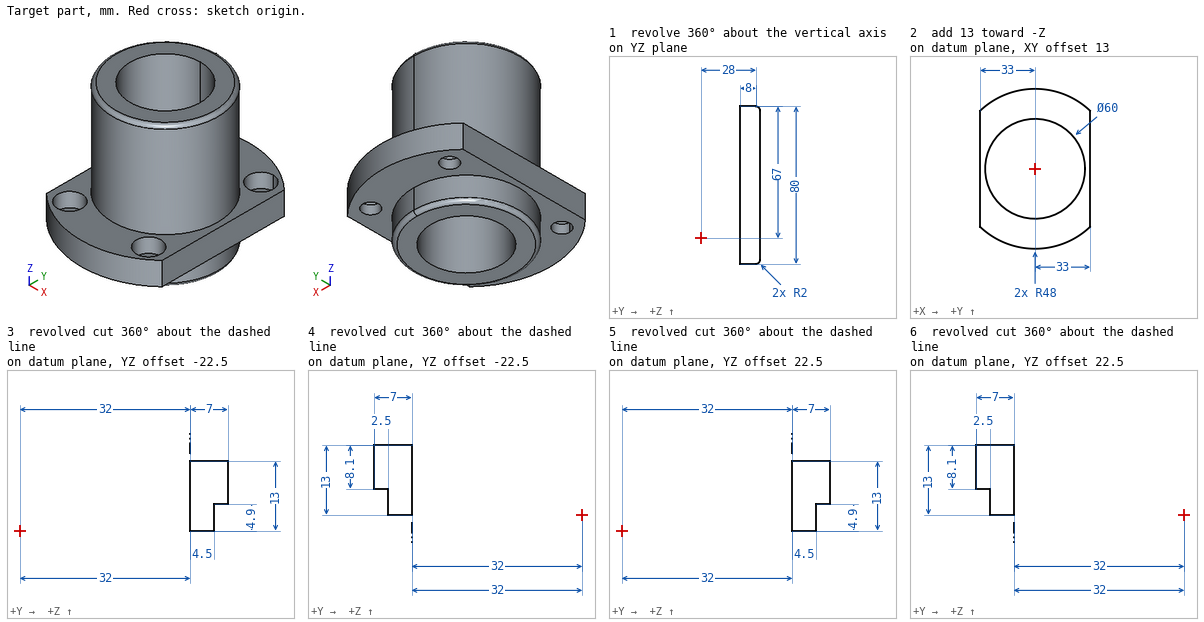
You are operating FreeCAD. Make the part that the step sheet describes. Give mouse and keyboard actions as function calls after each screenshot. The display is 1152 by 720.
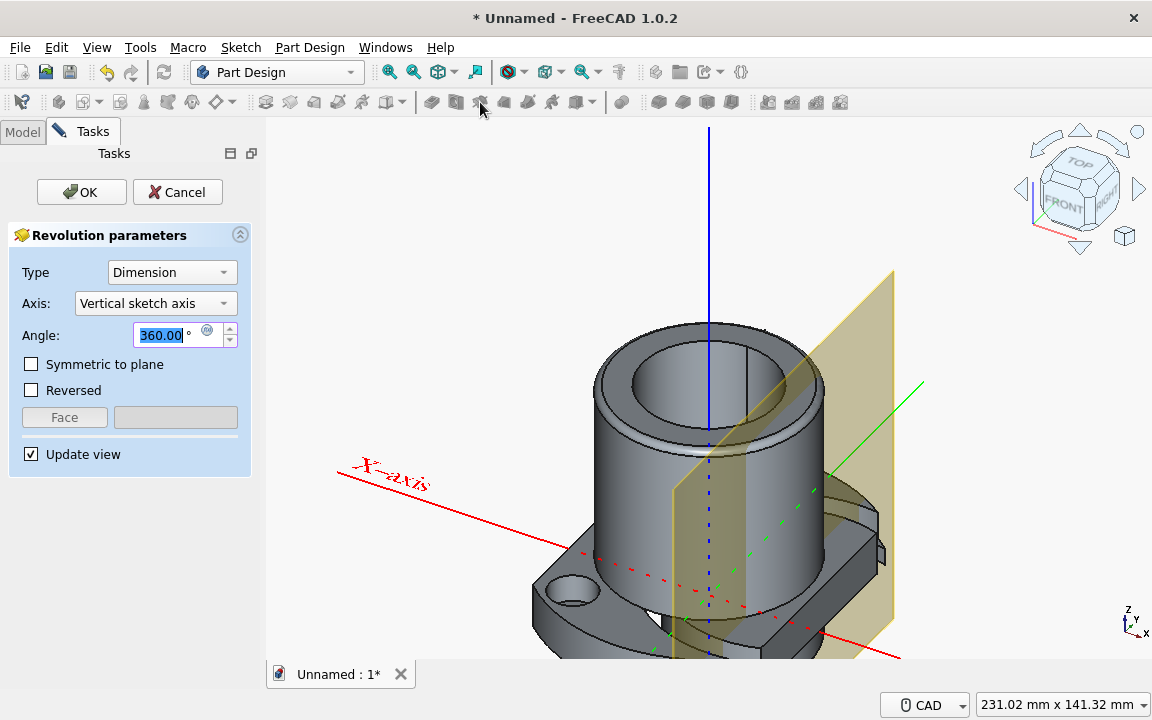
click(156, 304)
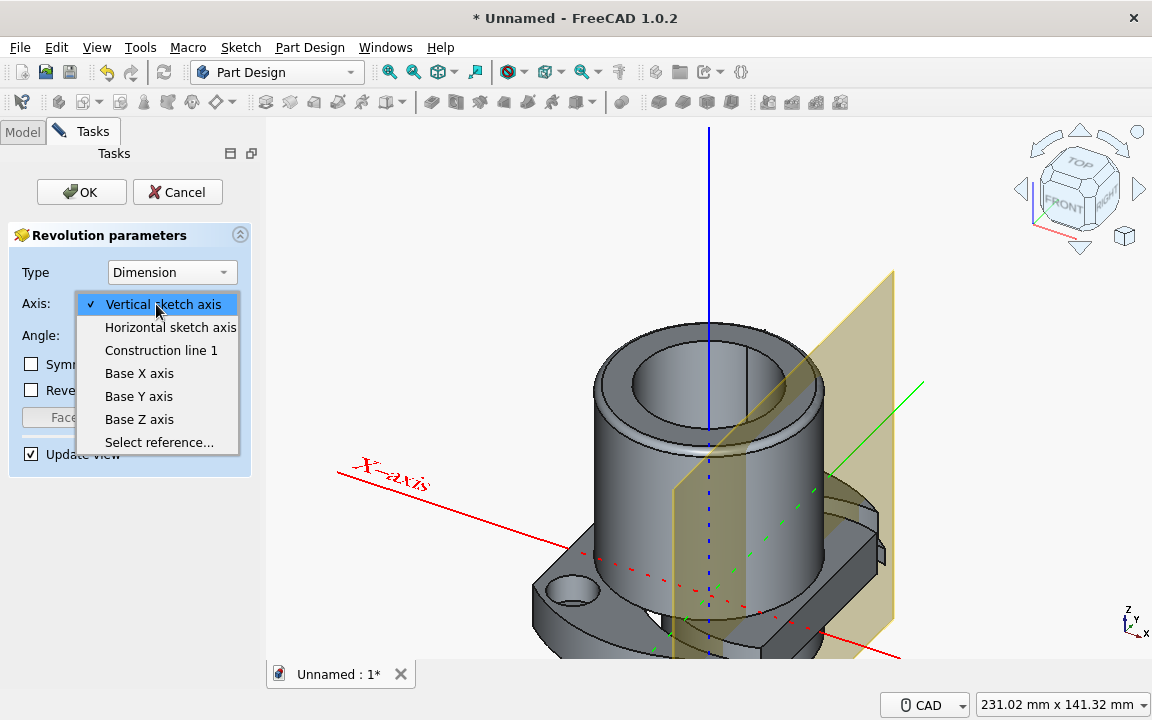
click(156, 350)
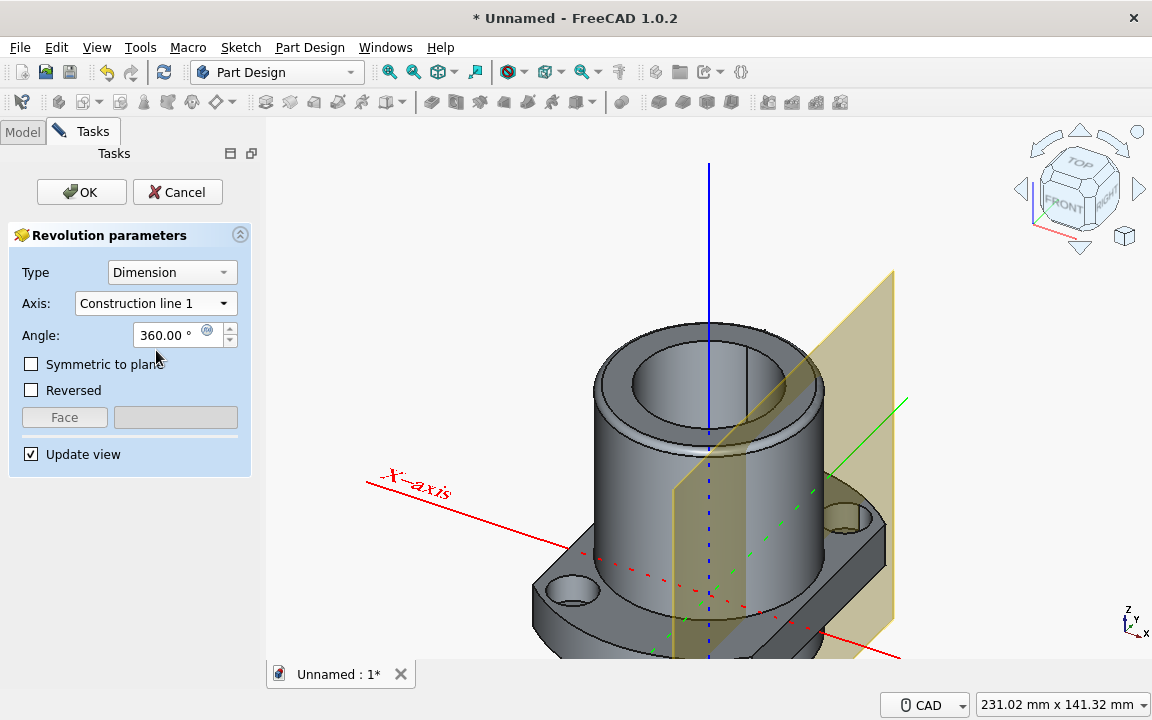
click(82, 192)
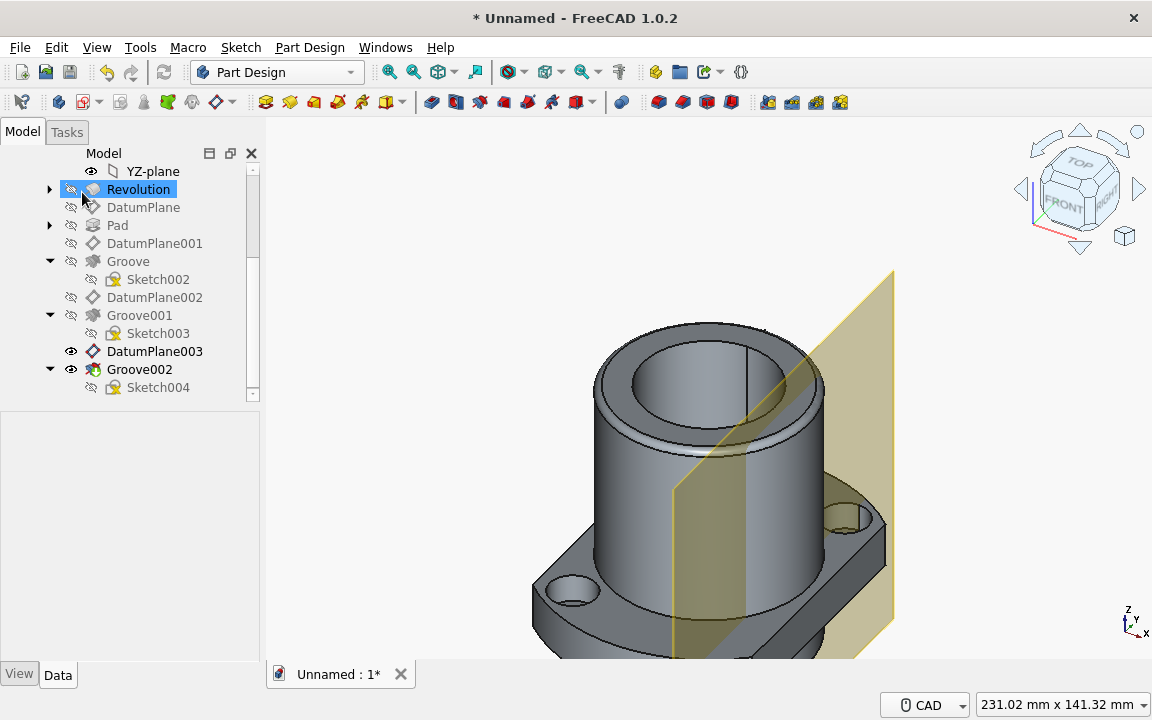
click(116, 351)
key(space)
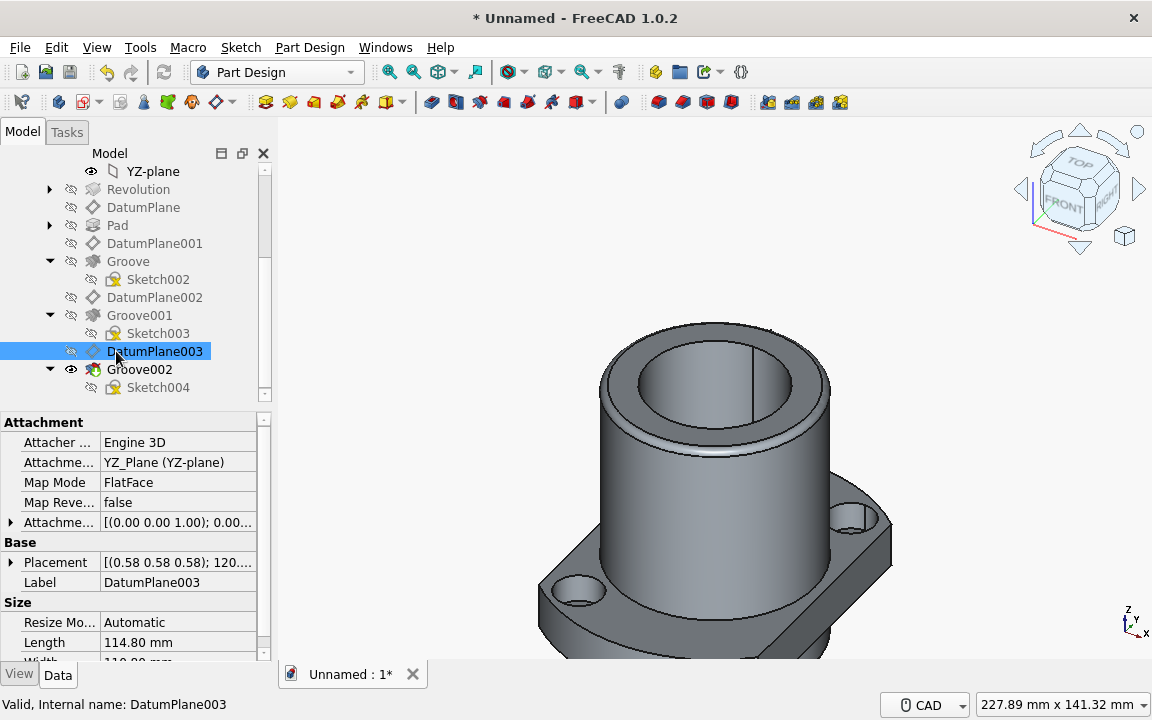
click(390, 72)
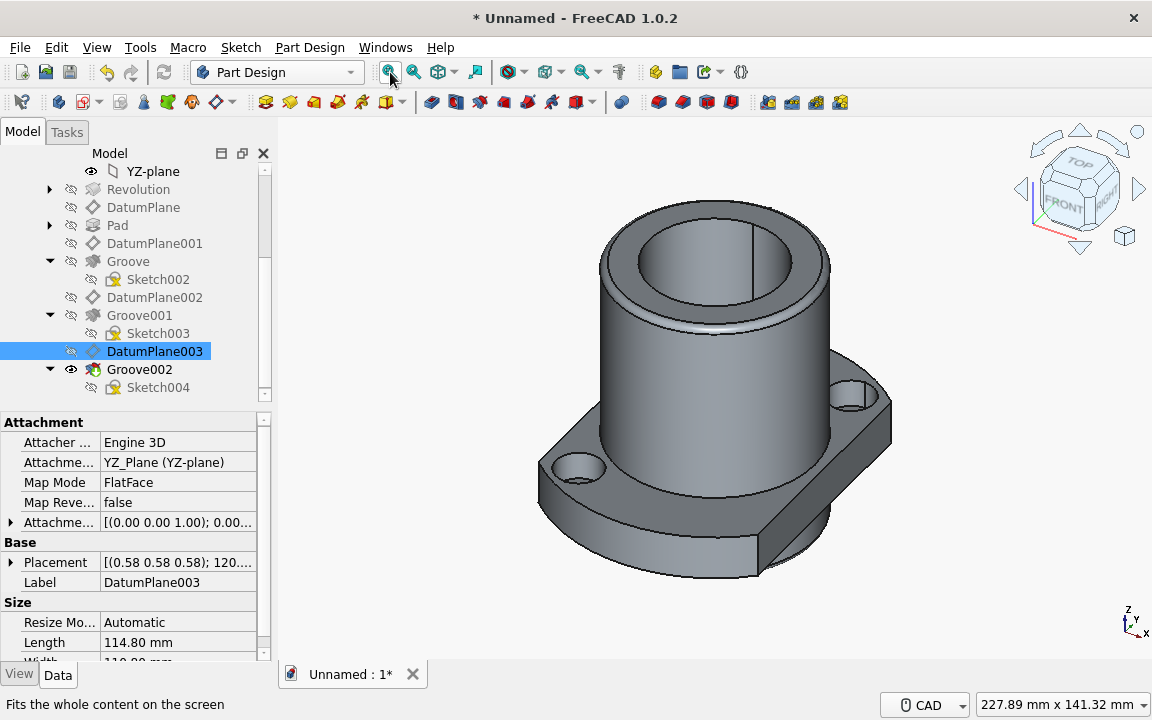
scroll(160, 275, down, 3)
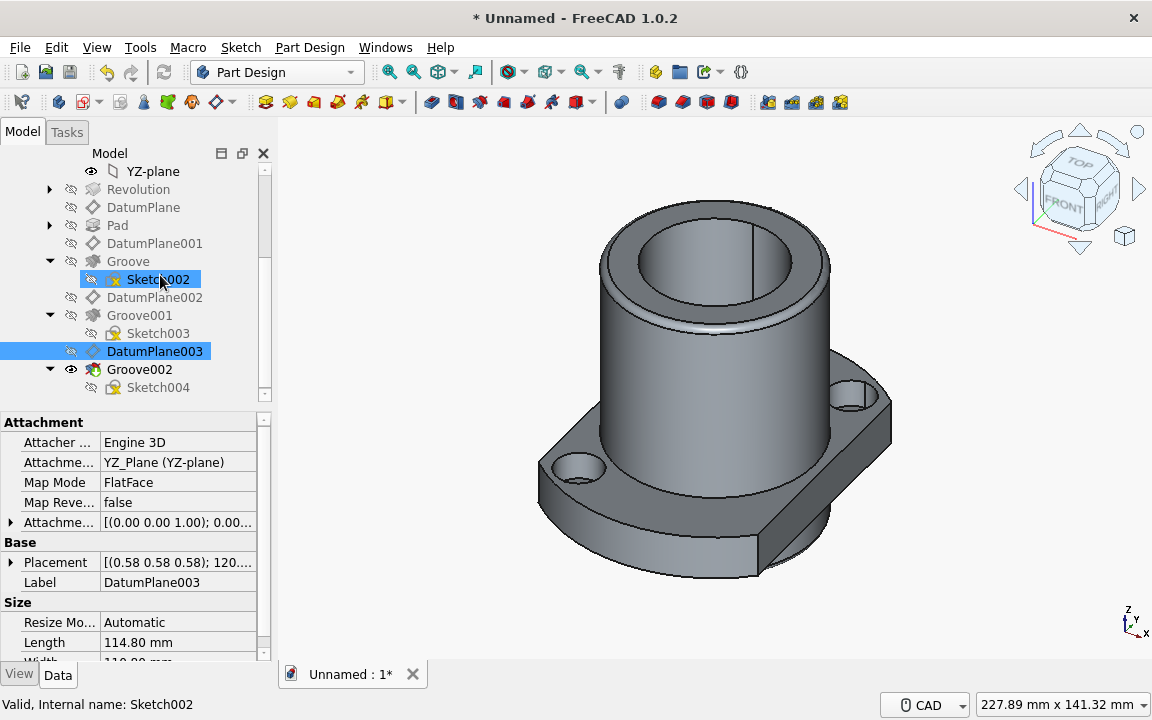
scroll(160, 275, up, 15)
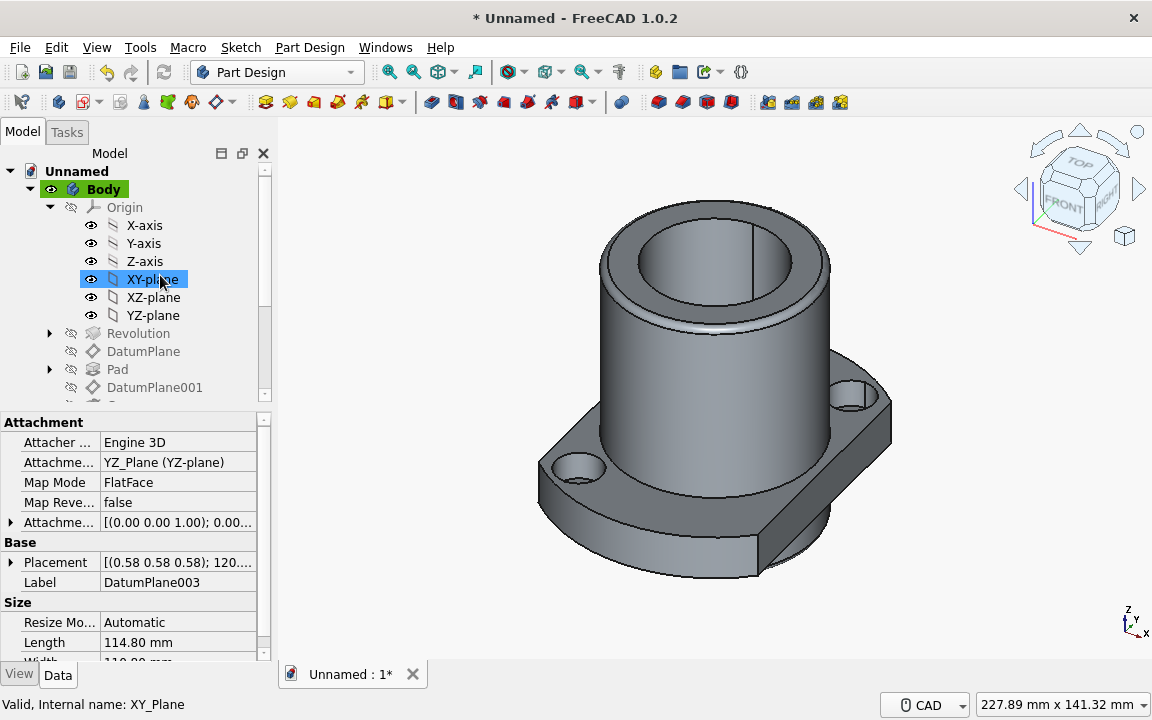
click(136, 315)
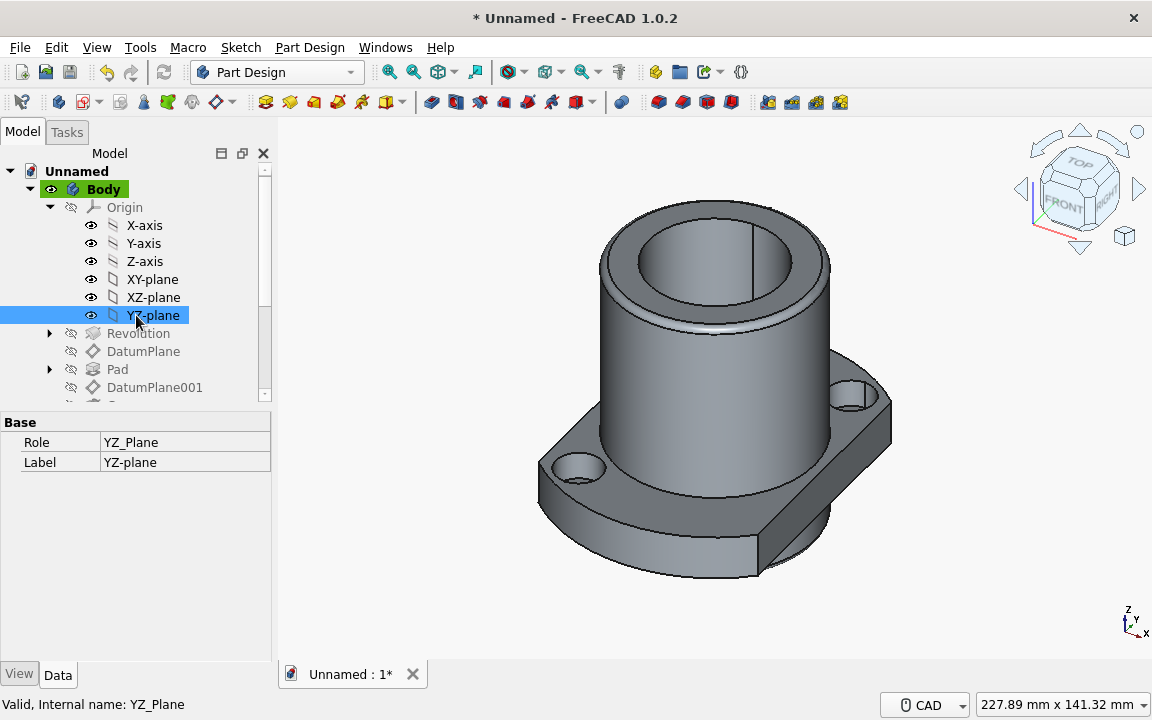
click(216, 102)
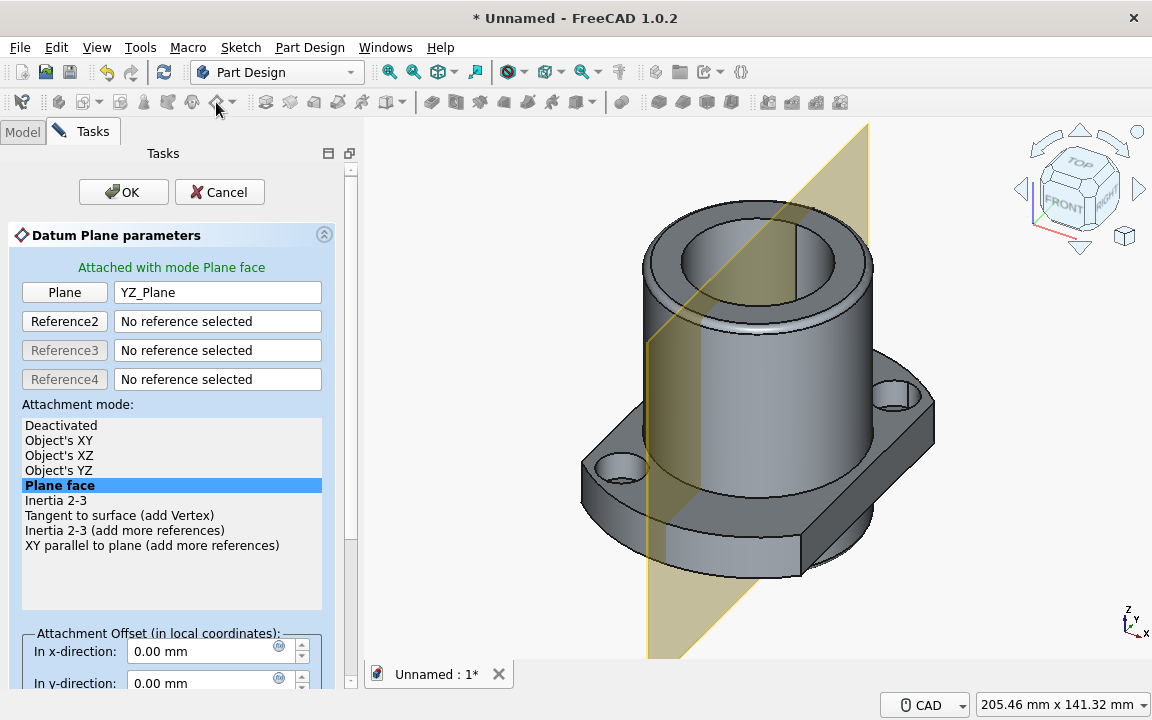
scroll(351, 426, down, 2)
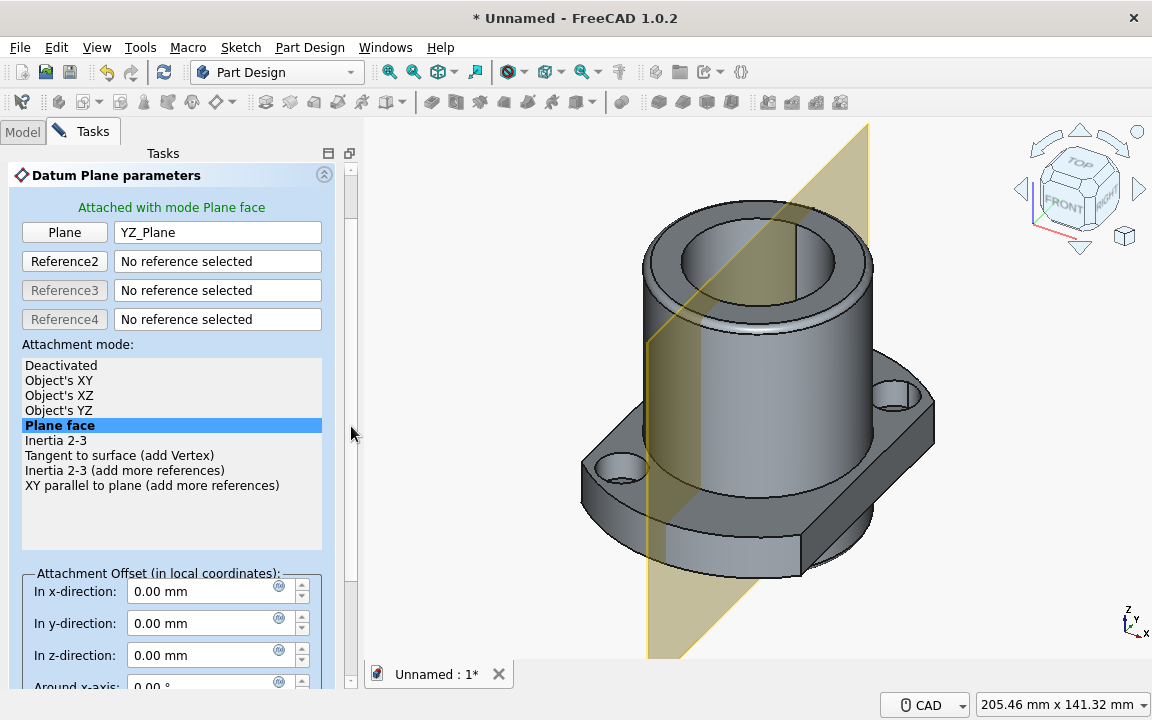
triple_click(210, 595)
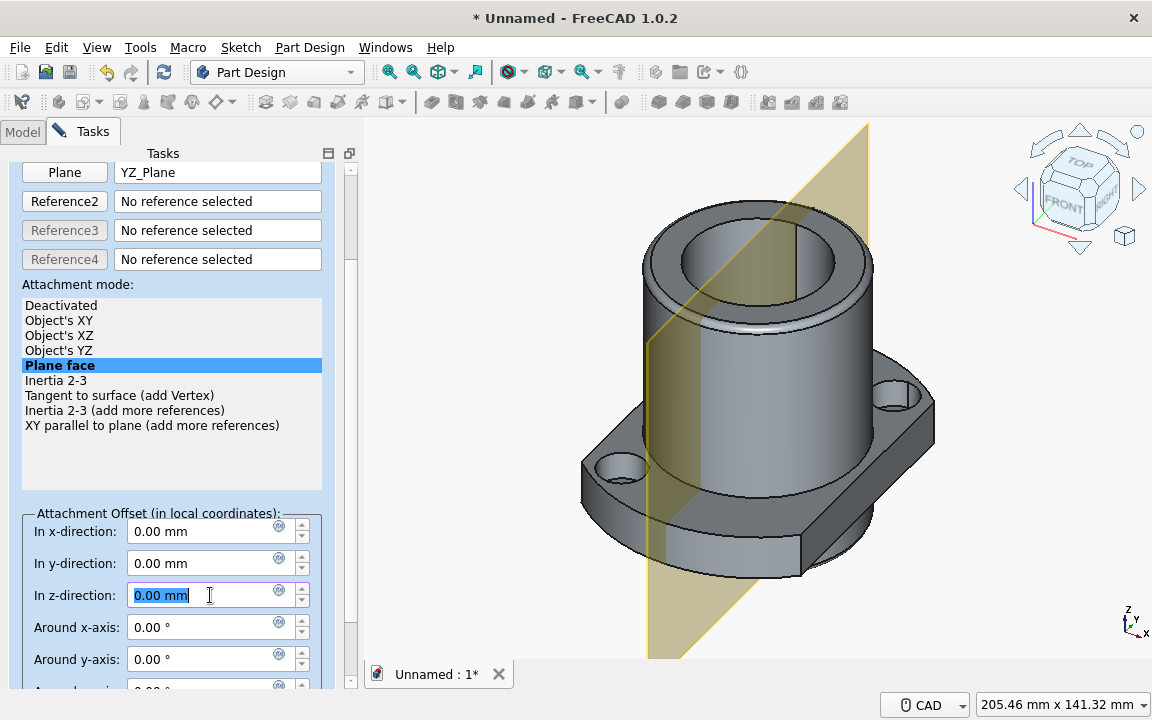
text(22.5)
key(Tab)